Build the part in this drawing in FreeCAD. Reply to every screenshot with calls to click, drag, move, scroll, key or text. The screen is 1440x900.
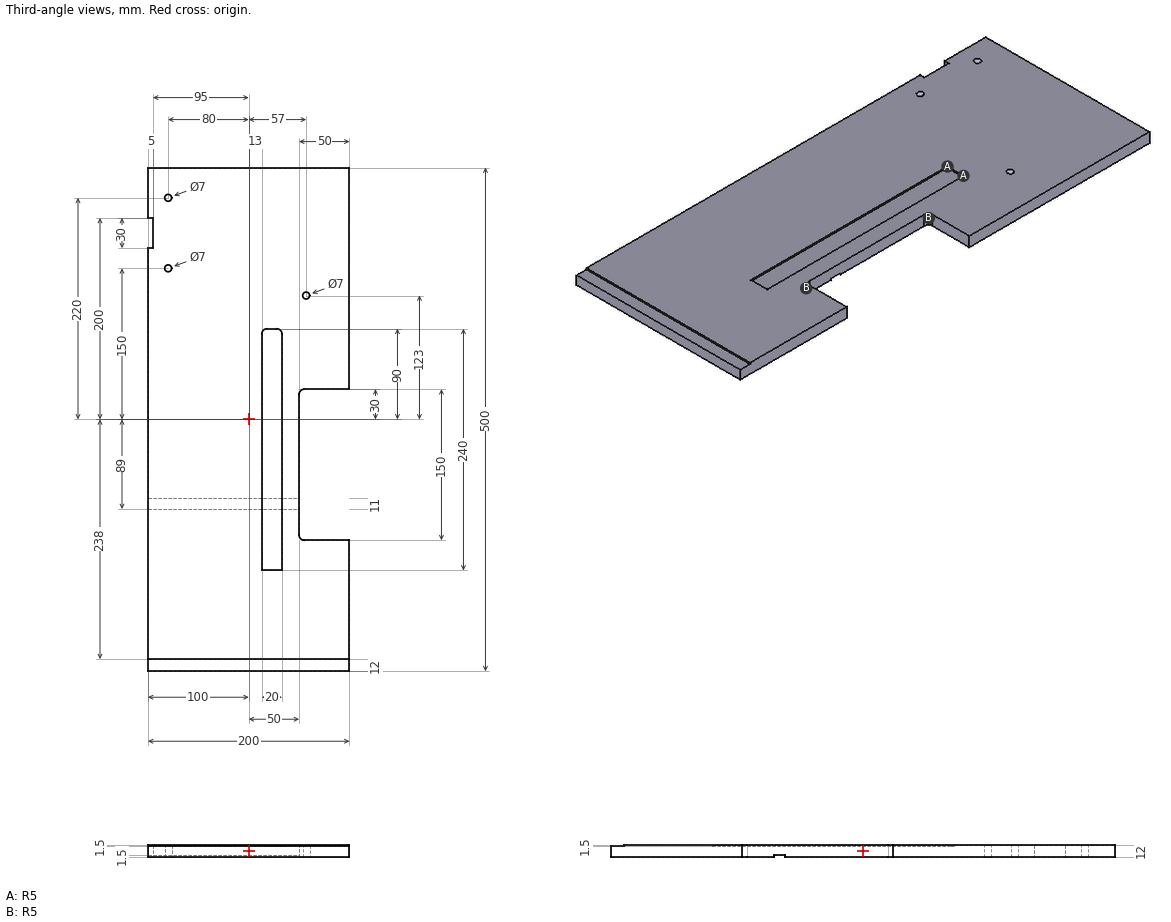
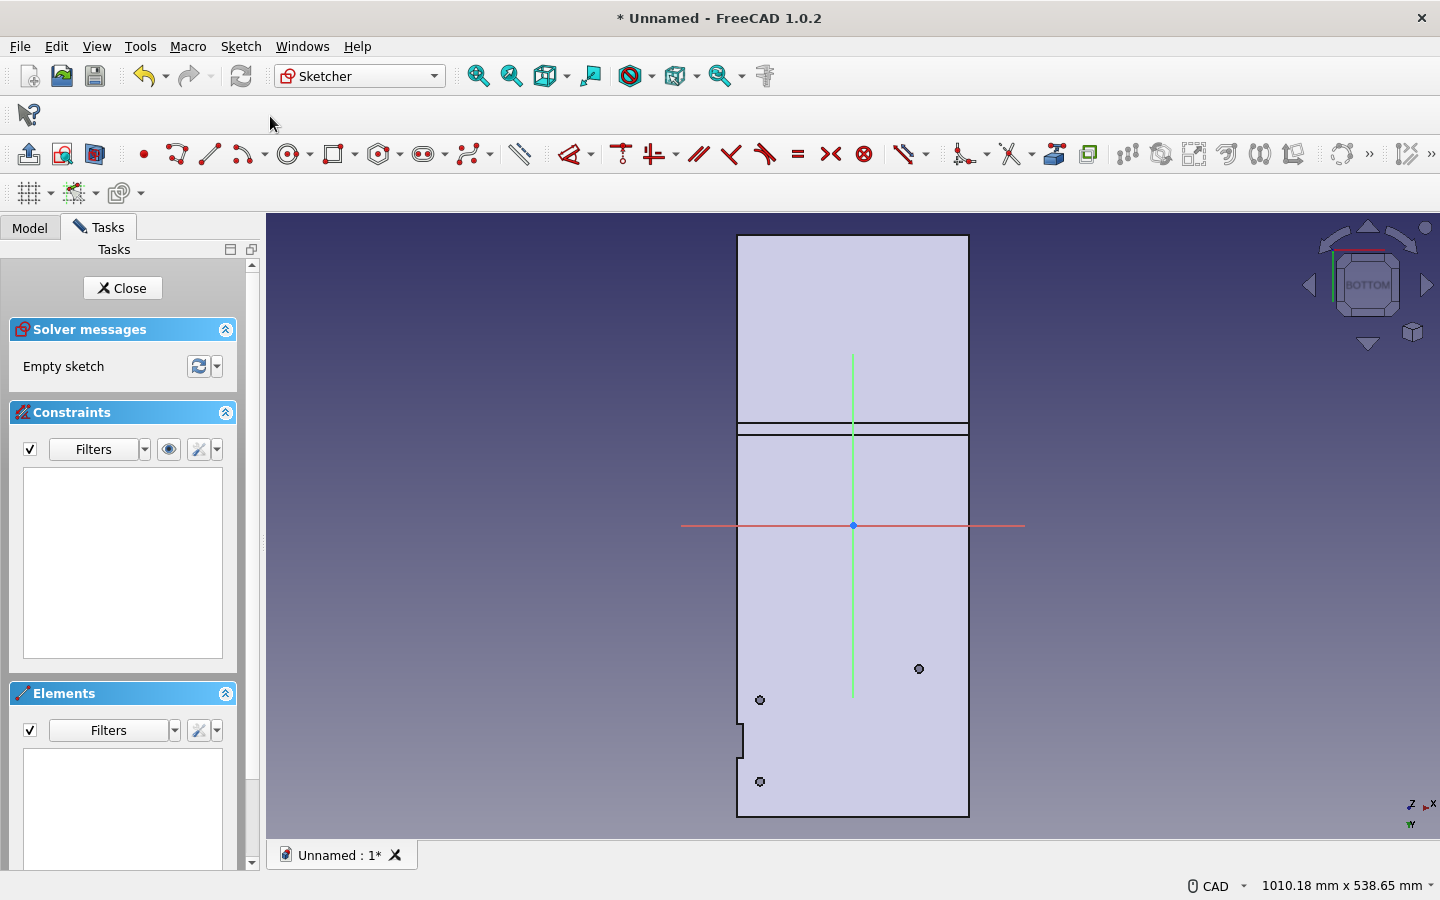
scroll(1014, 431, up, 4)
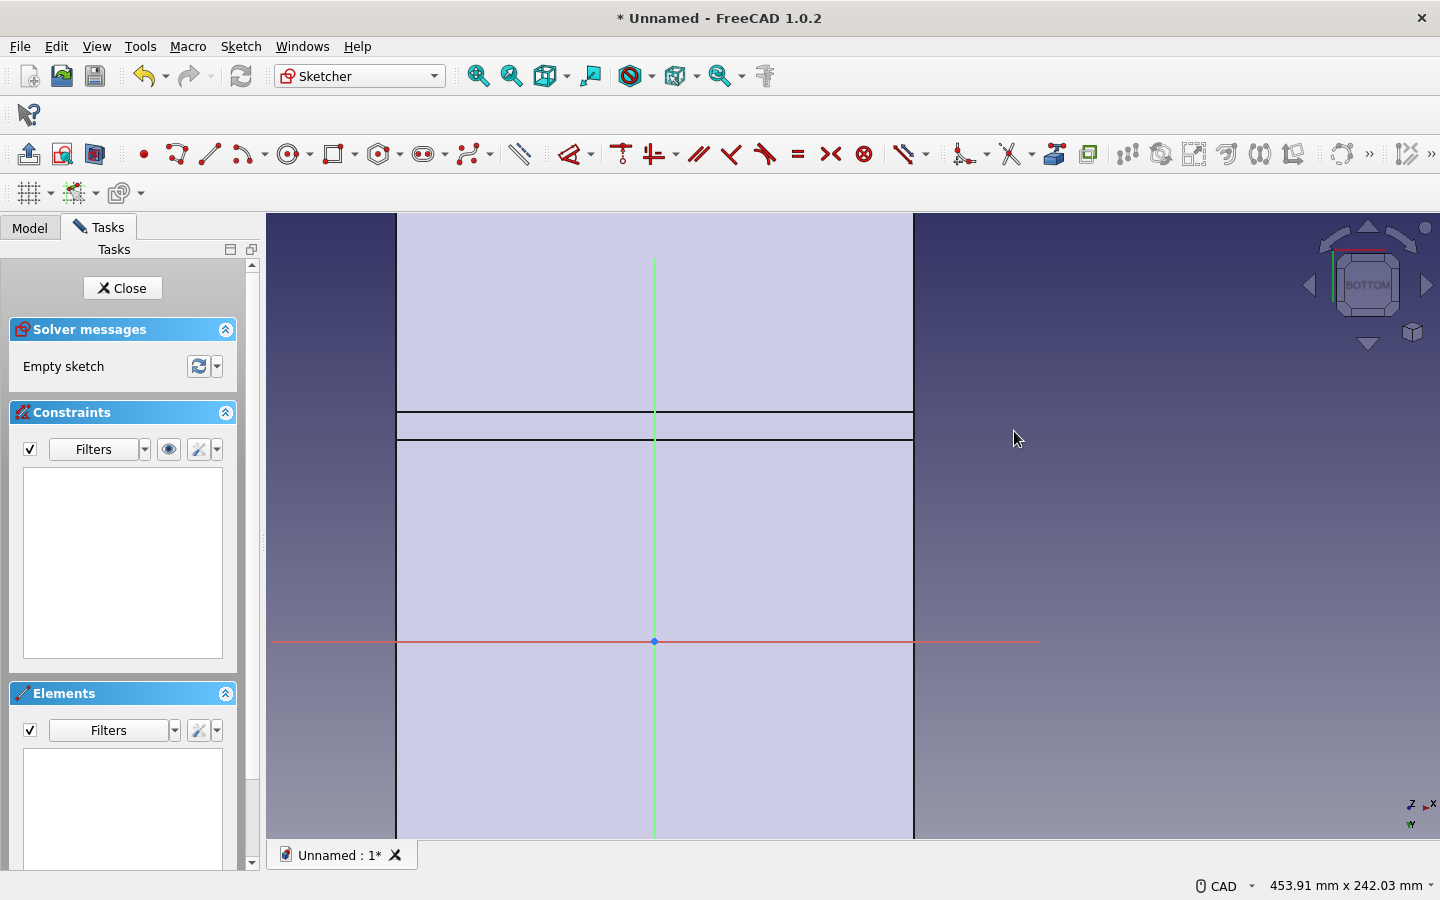
click(332, 154)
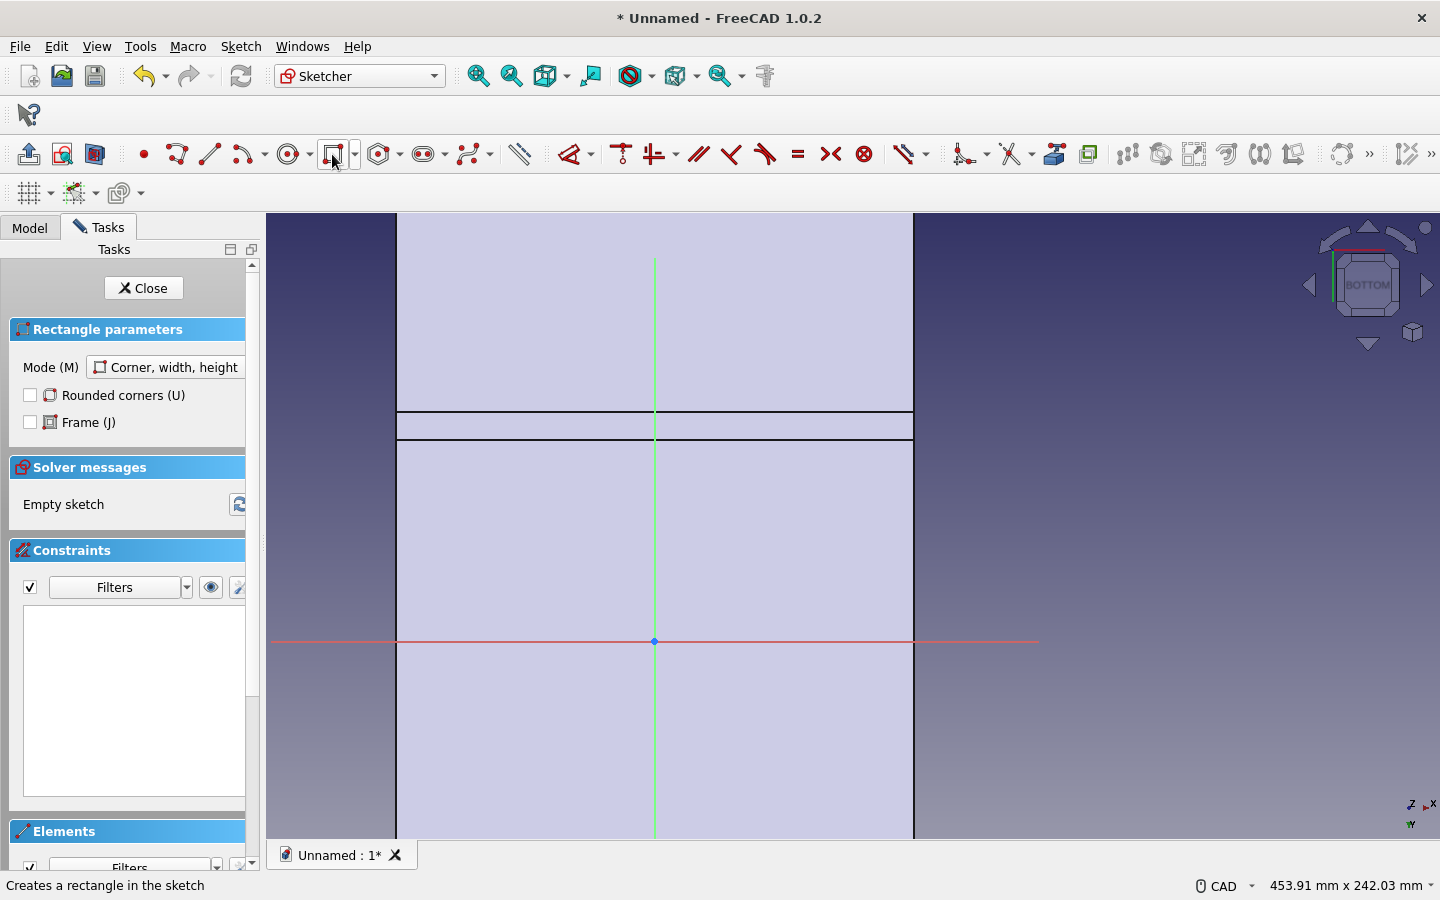
click(784, 332)
move(914, 720)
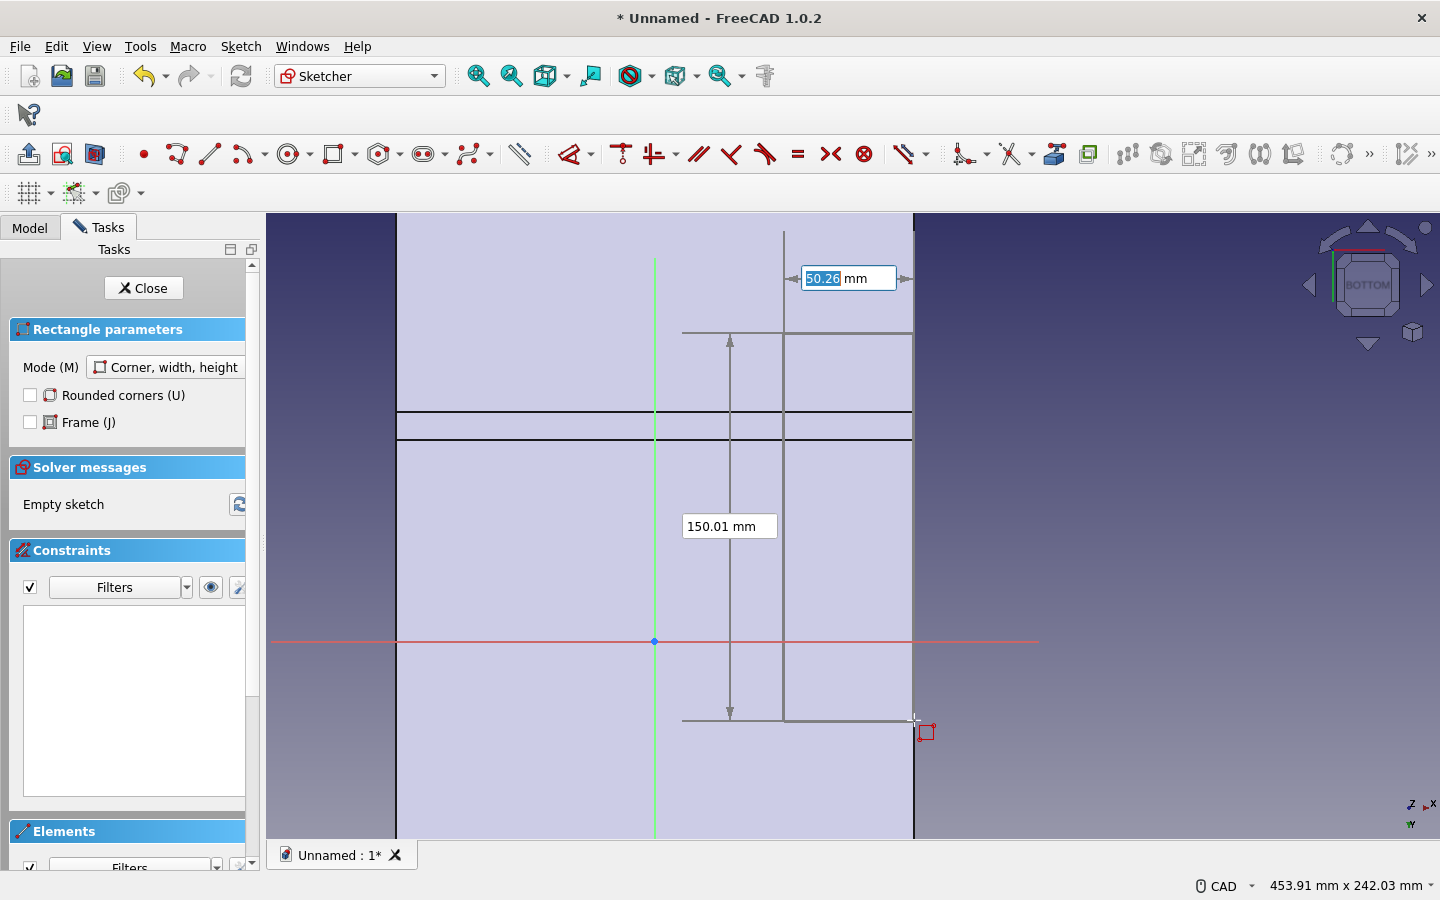
text(50)
key(Tab)
text(150)
key(Return)
key(Escape)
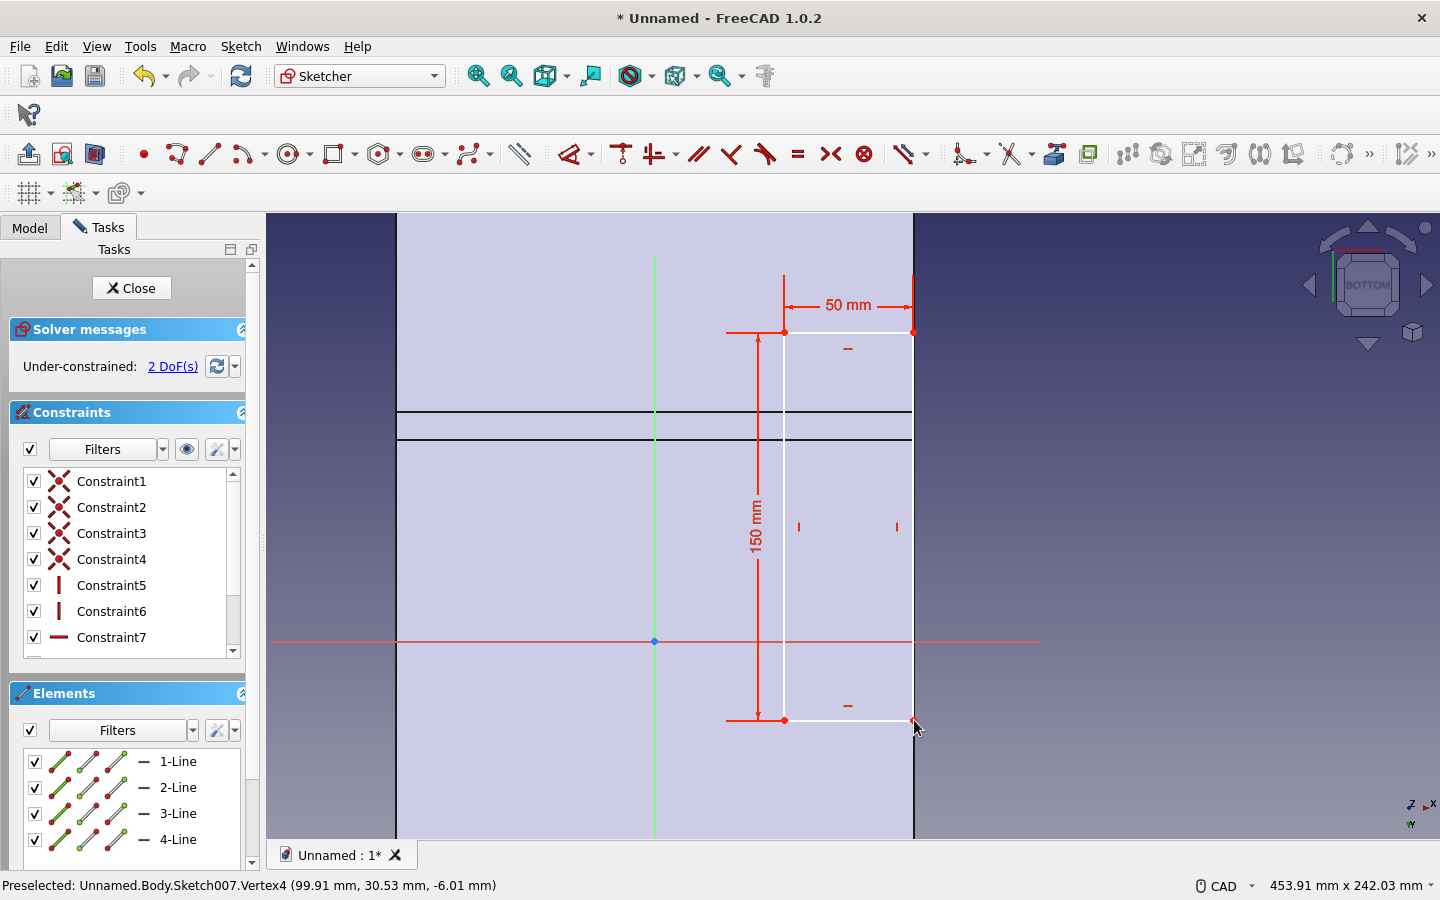
click(568, 154)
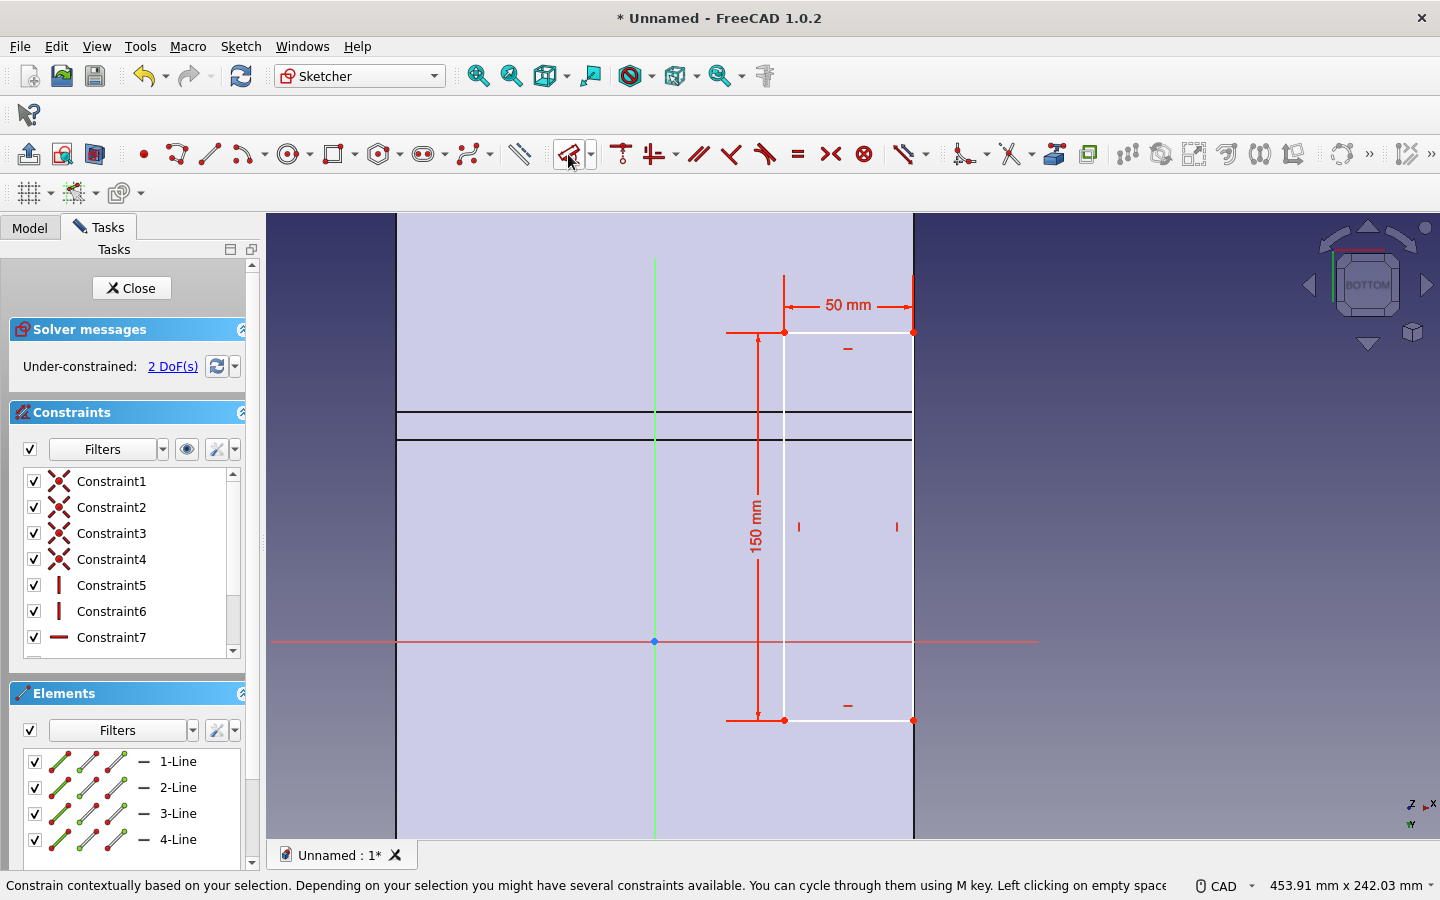
click(784, 333)
click(719, 299)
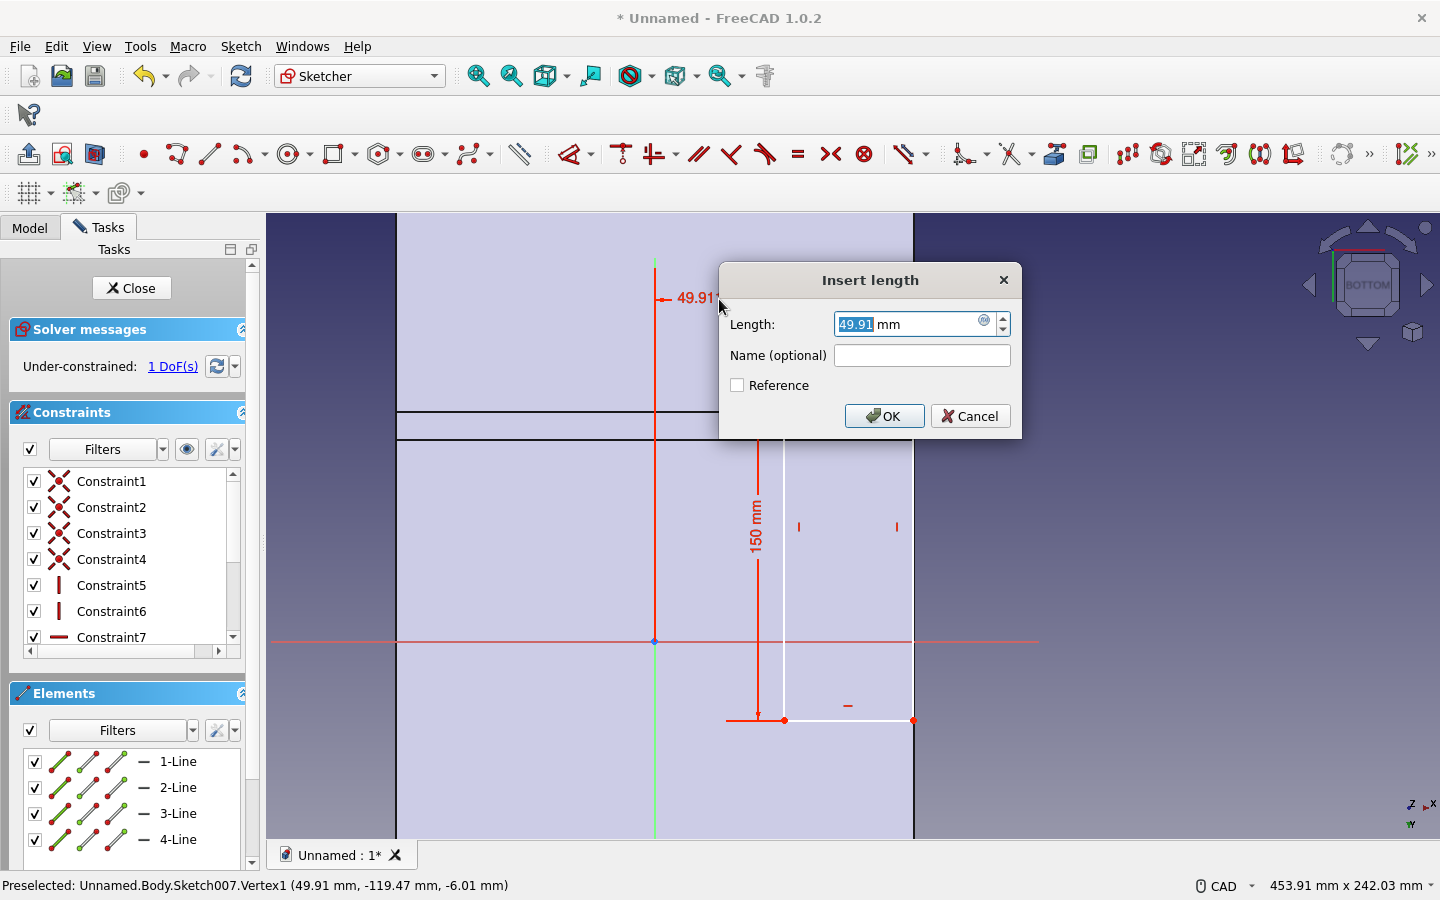
text(50)
key(Return)